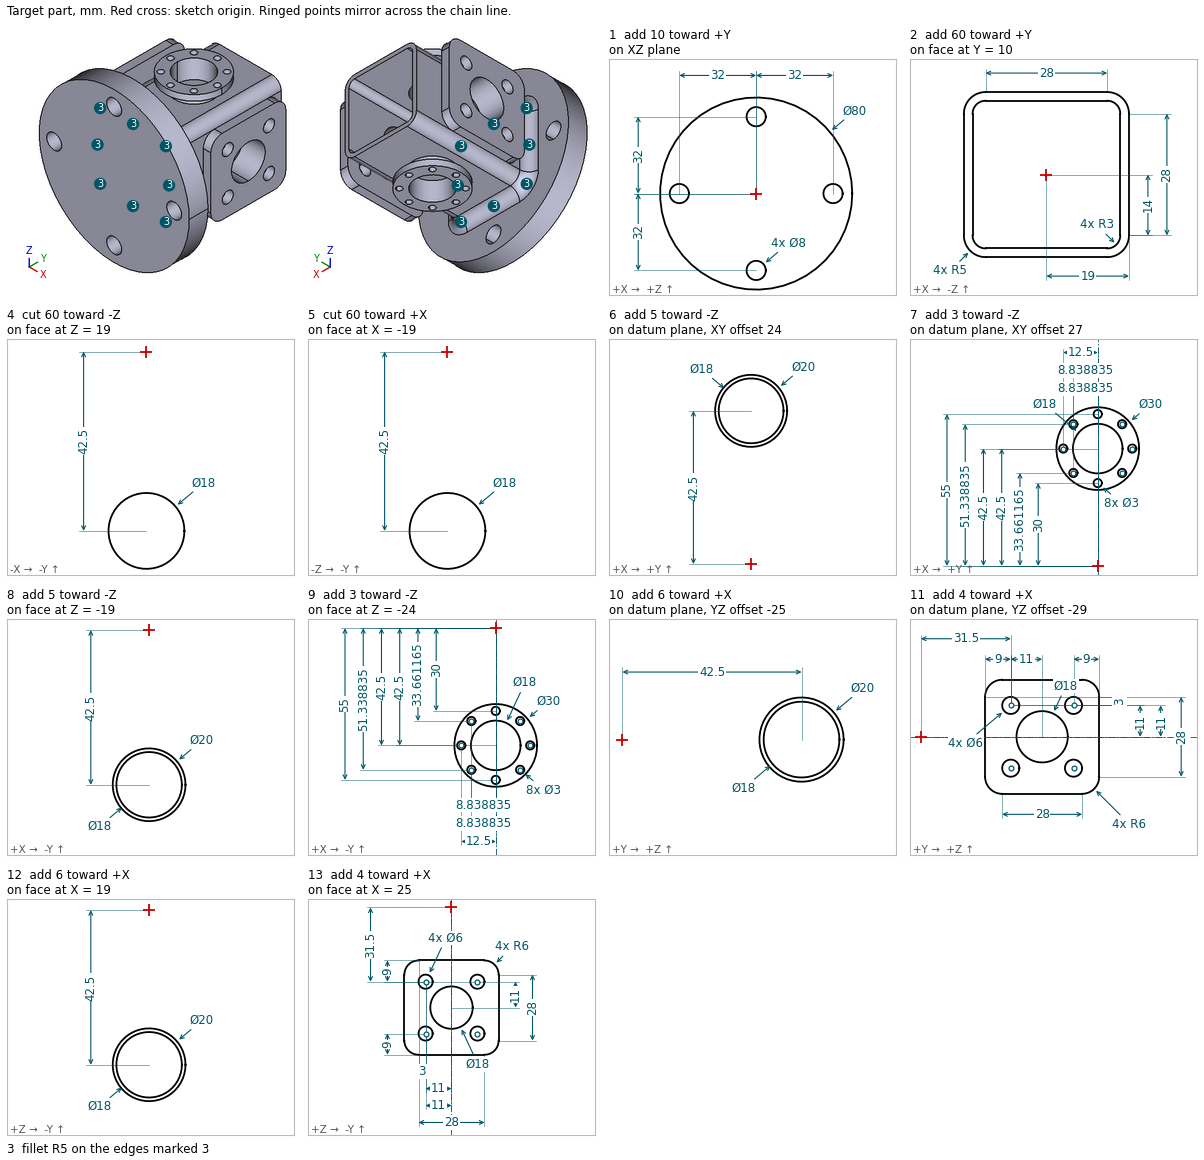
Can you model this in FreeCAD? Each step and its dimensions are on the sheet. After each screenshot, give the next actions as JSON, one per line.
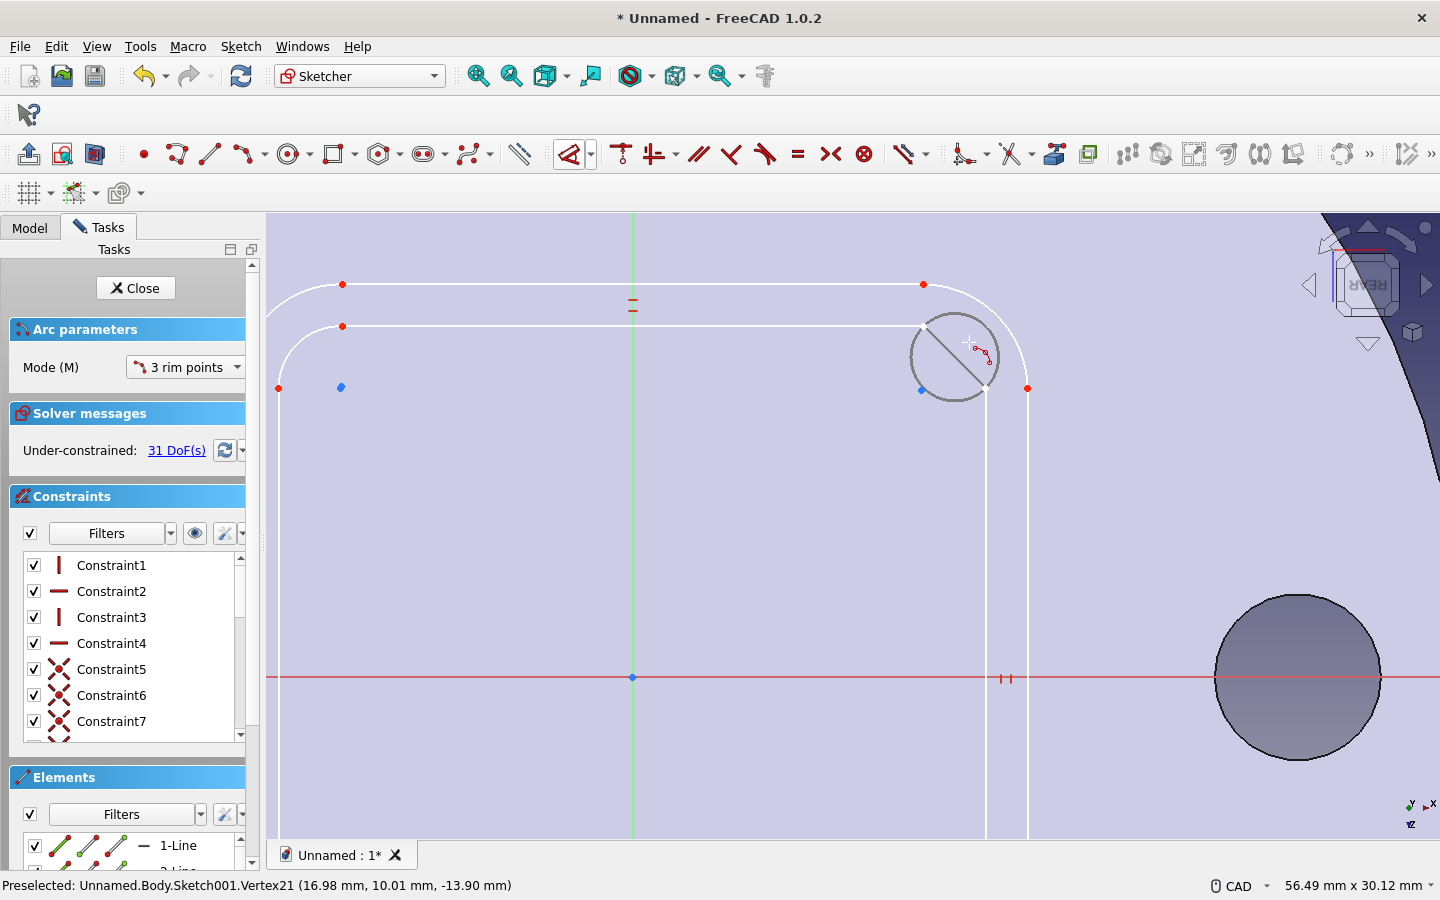
{"action": "left_click", "coordinate": [968, 342]}
{"action": "key", "text": "Escape"}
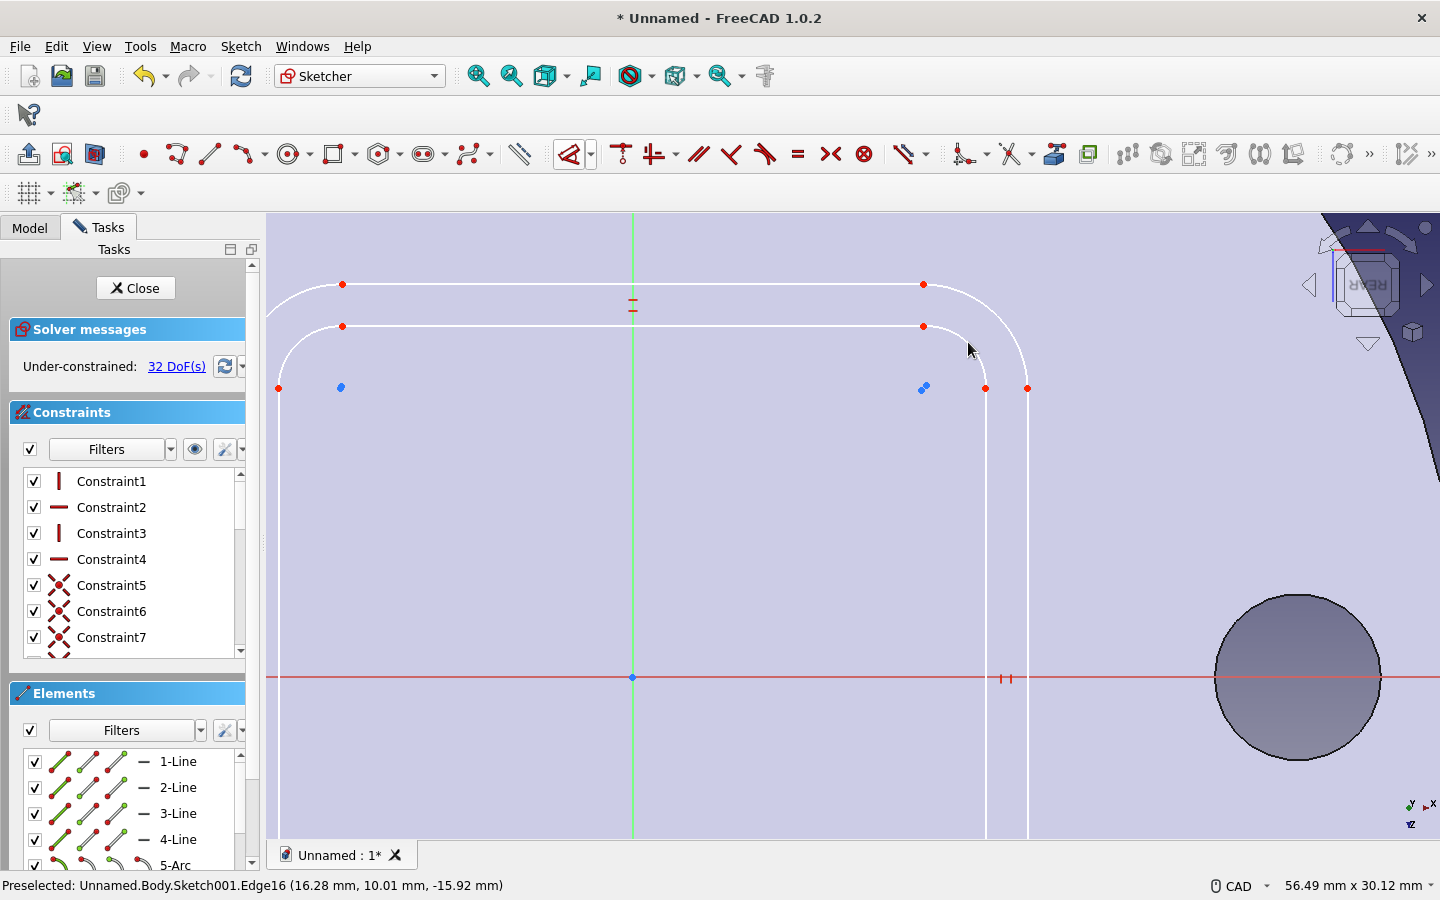
{"action": "left_click", "coordinate": [1028, 795]}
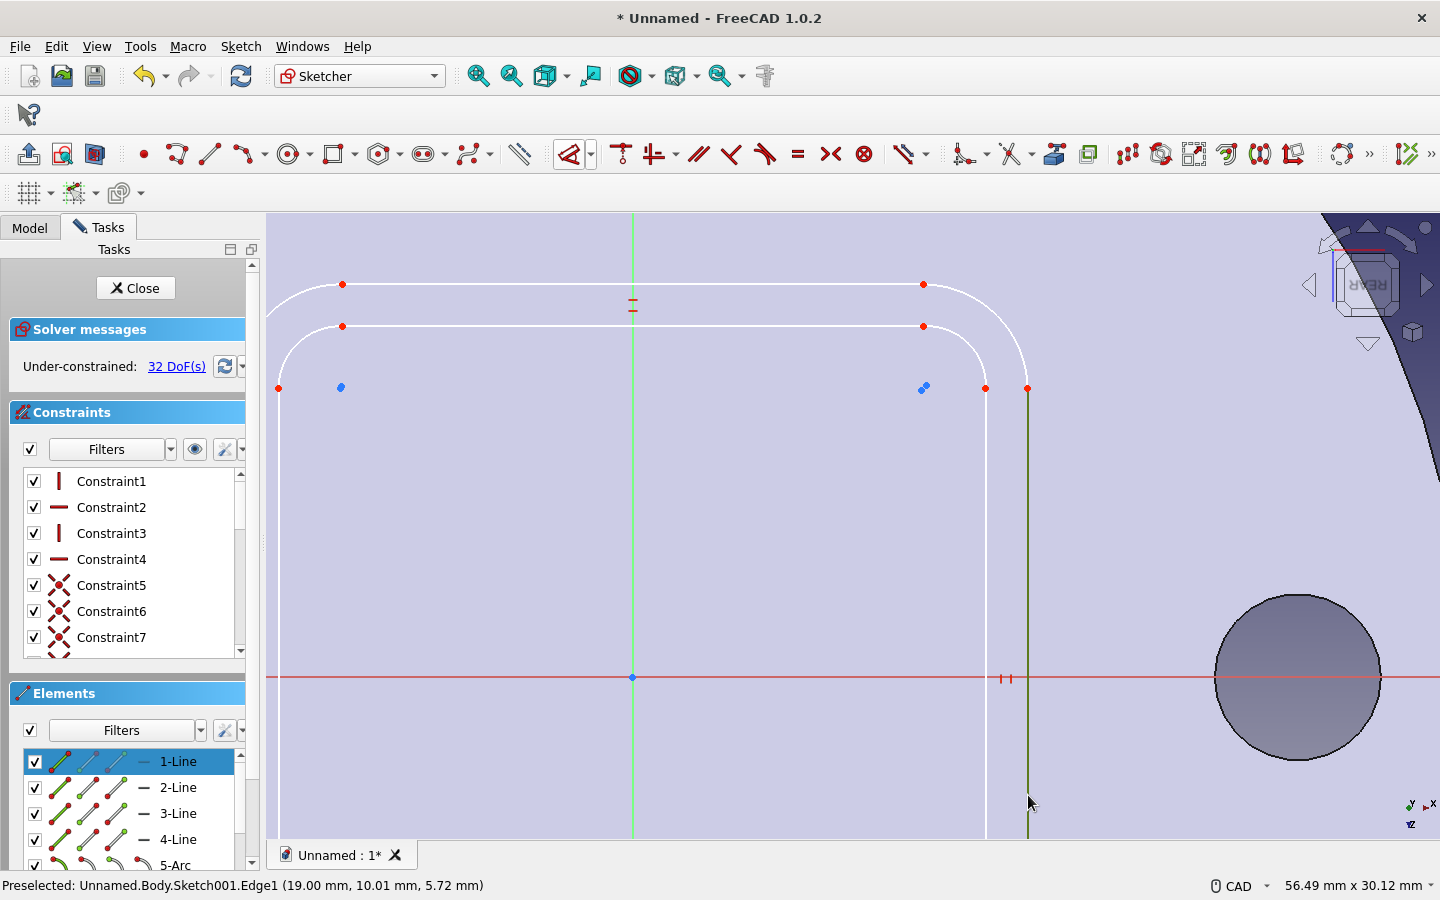
{"action": "left_click", "coordinate": [1016, 341]}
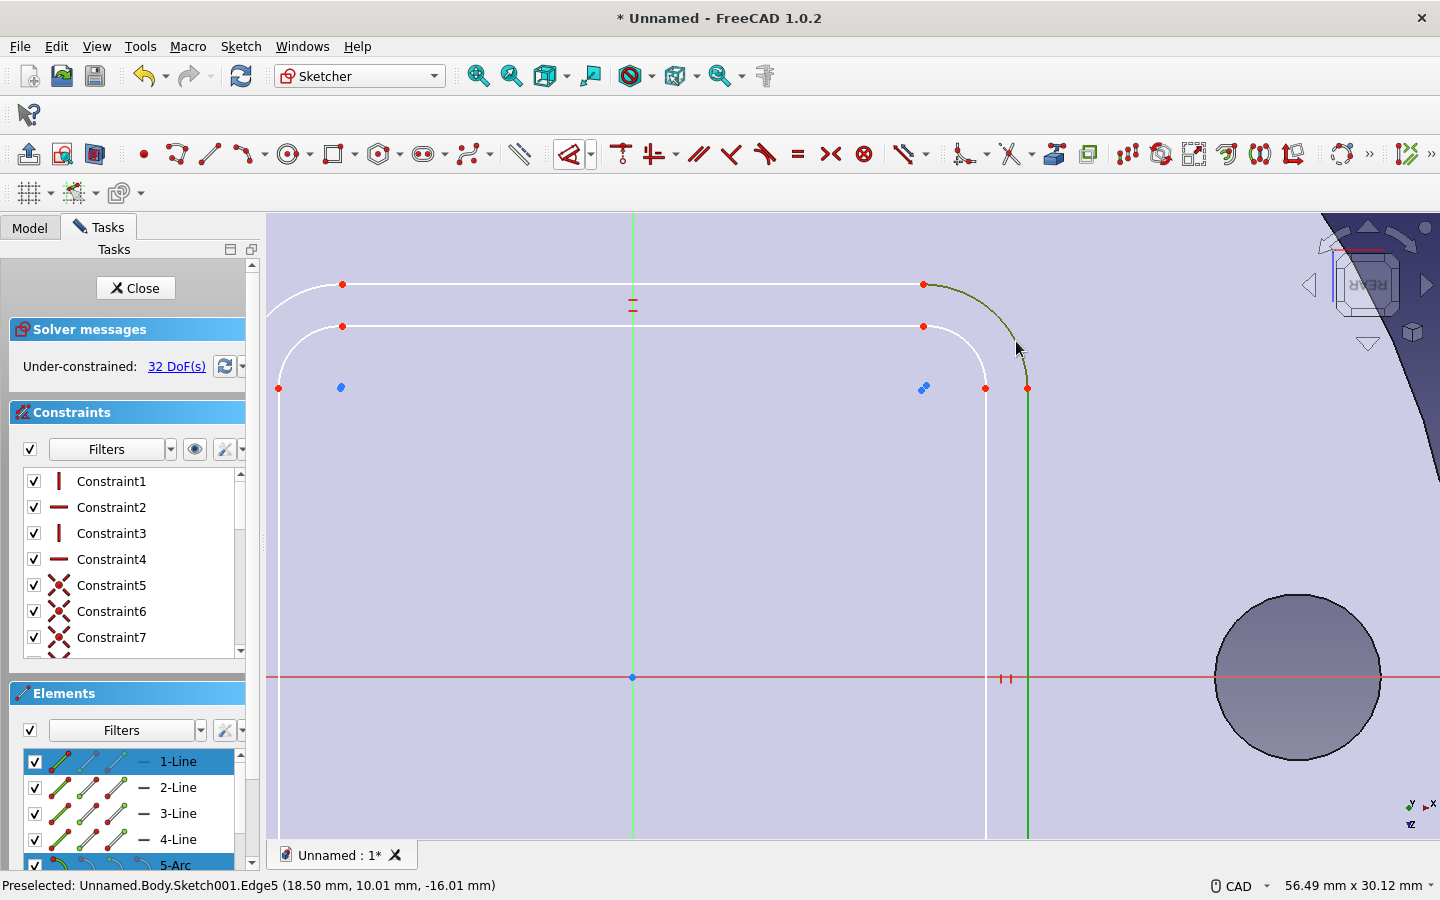
{"action": "key", "text": "t"}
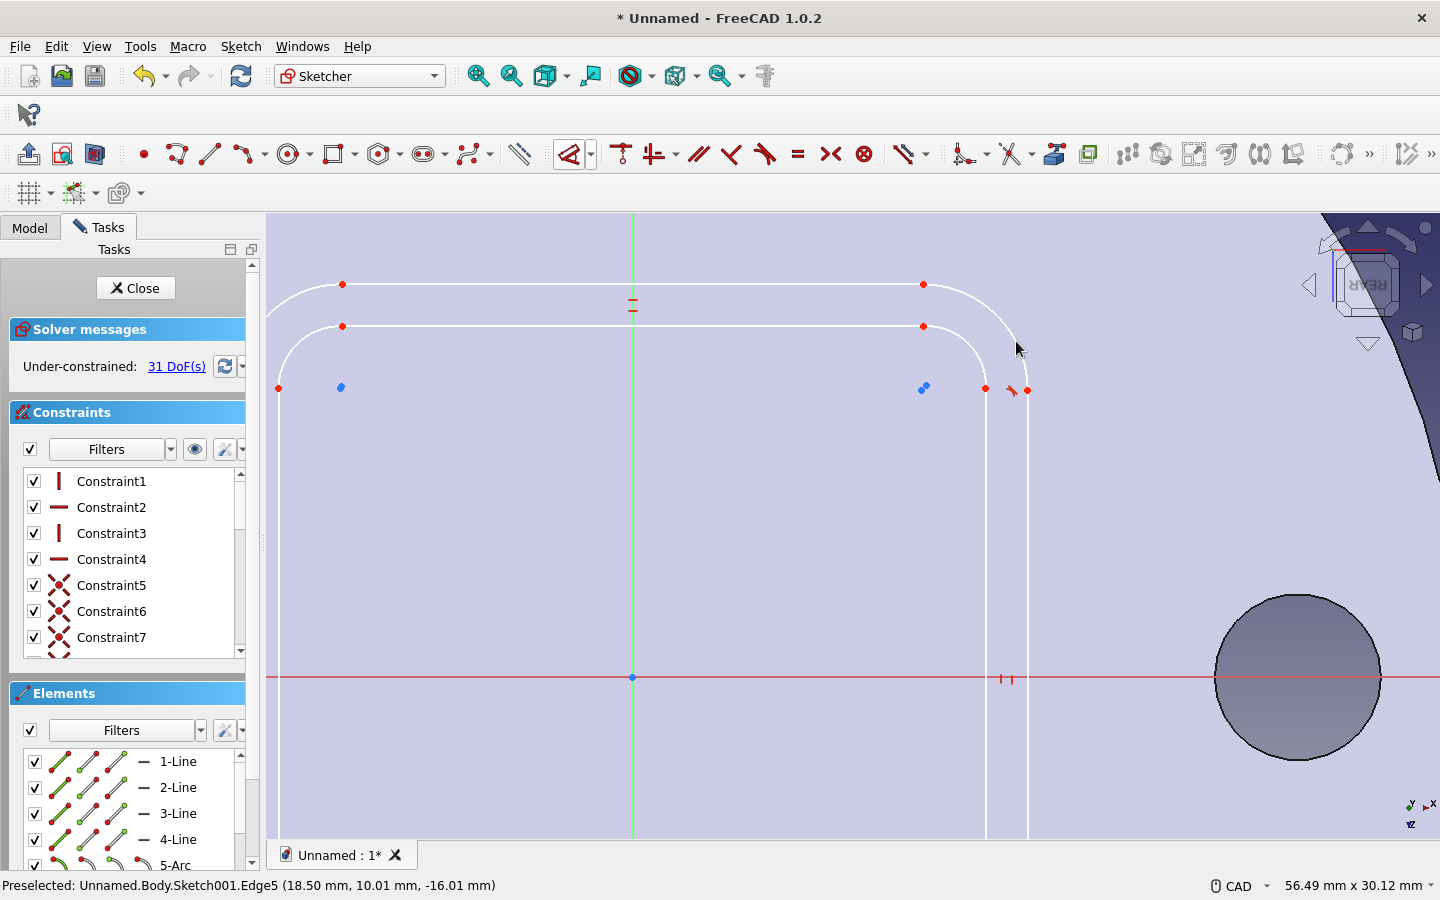
{"action": "left_click", "coordinate": [1028, 796]}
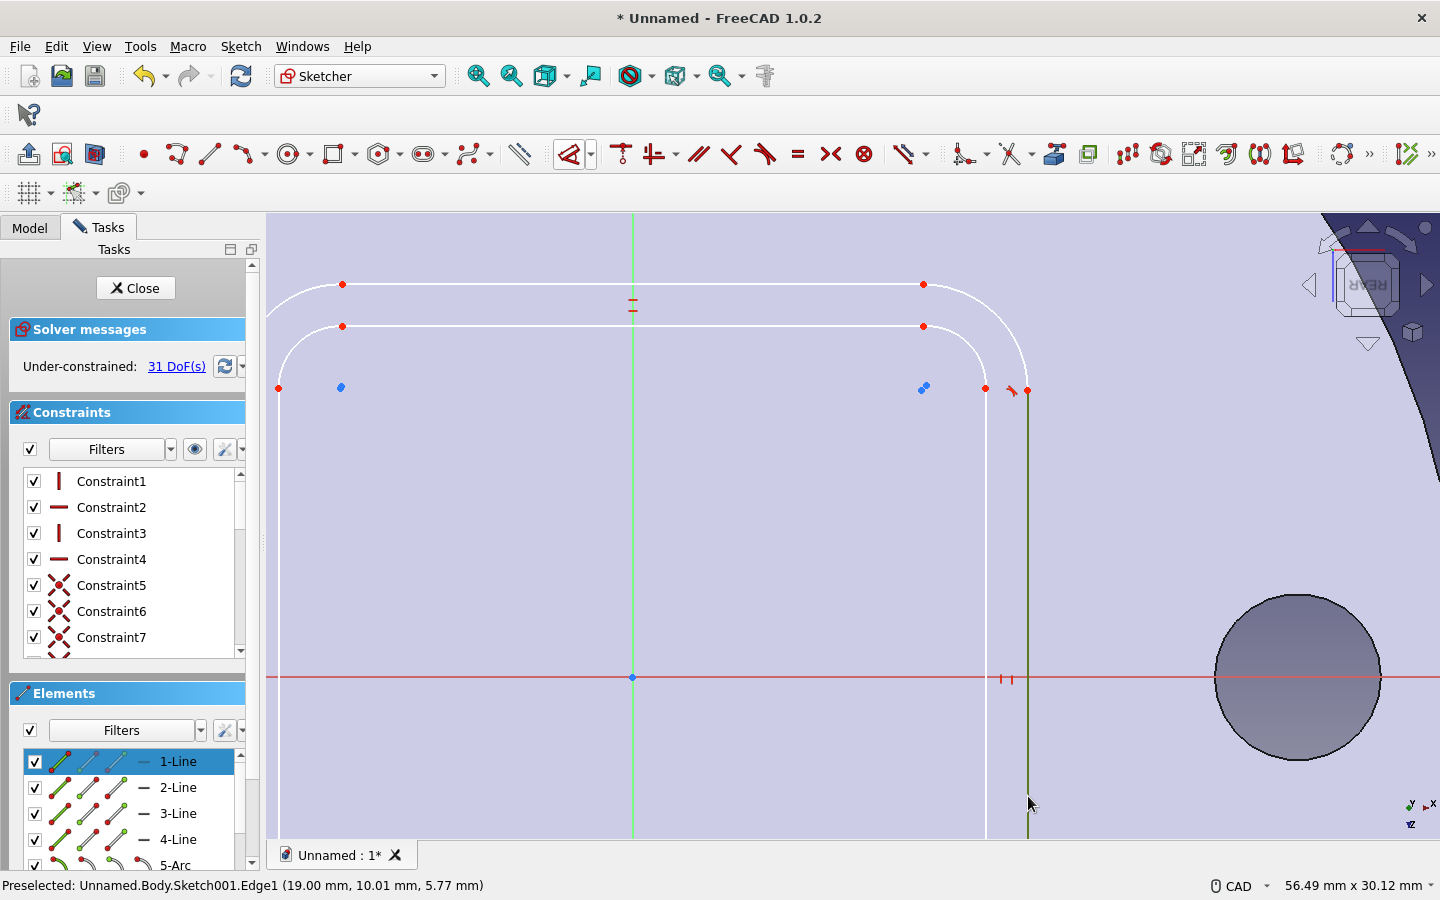
{"action": "scroll", "coordinate": [969, 342], "scroll_direction": "down", "scroll_amount": 3}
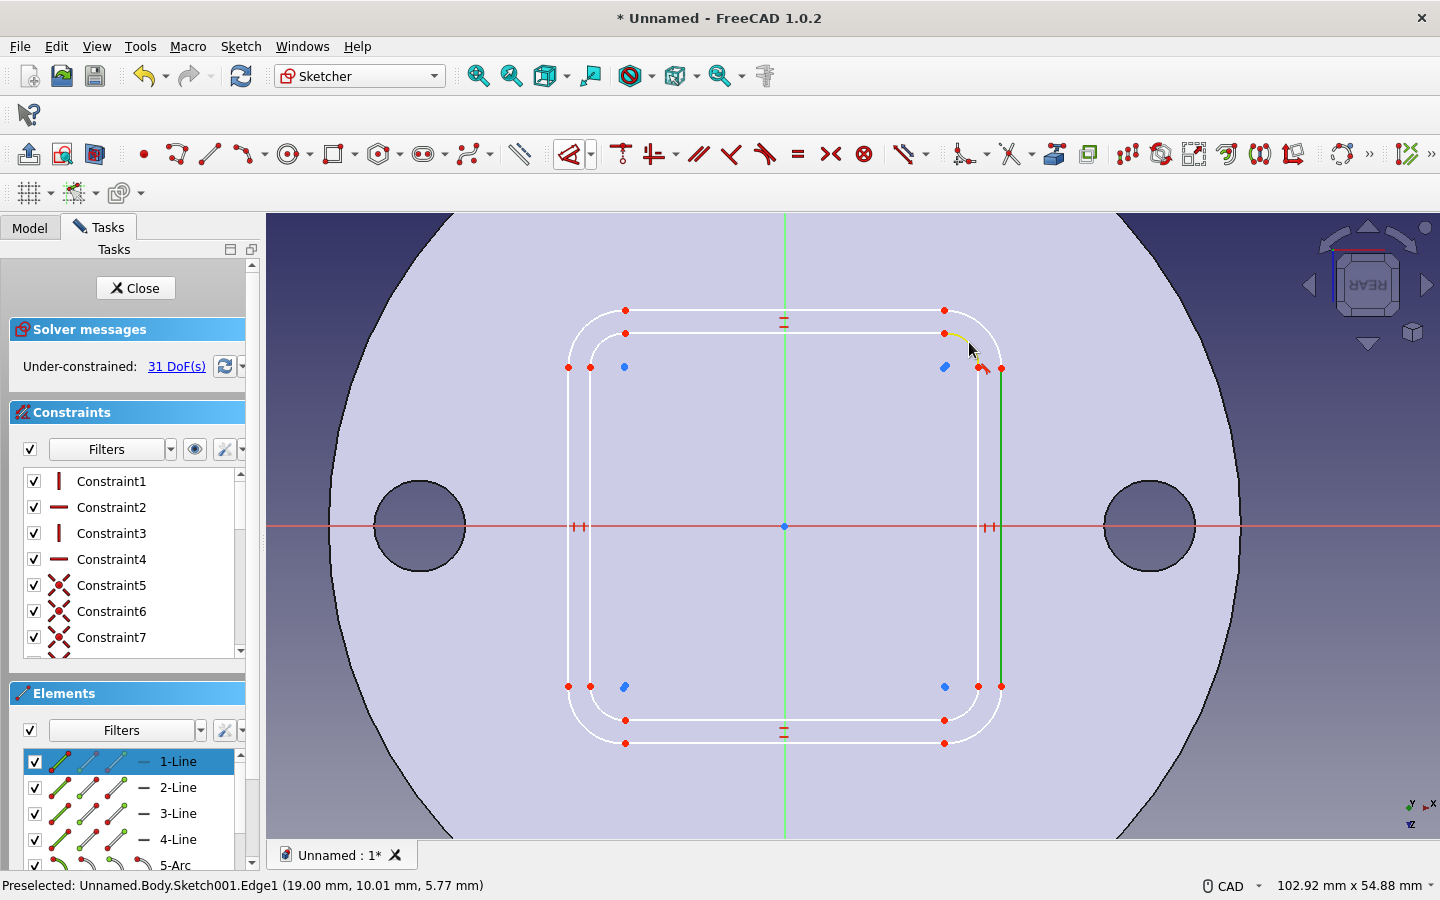
{"action": "left_click", "coordinate": [970, 737]}